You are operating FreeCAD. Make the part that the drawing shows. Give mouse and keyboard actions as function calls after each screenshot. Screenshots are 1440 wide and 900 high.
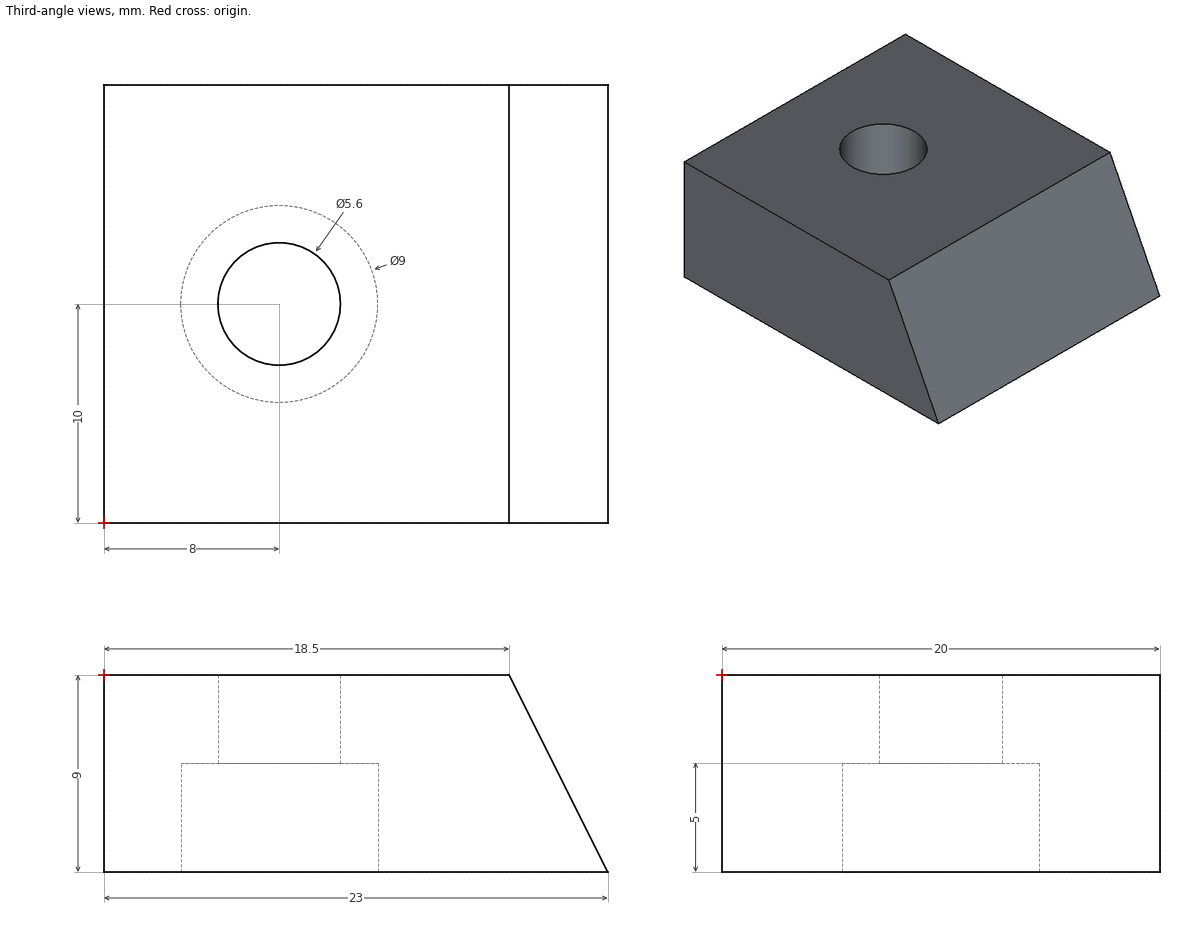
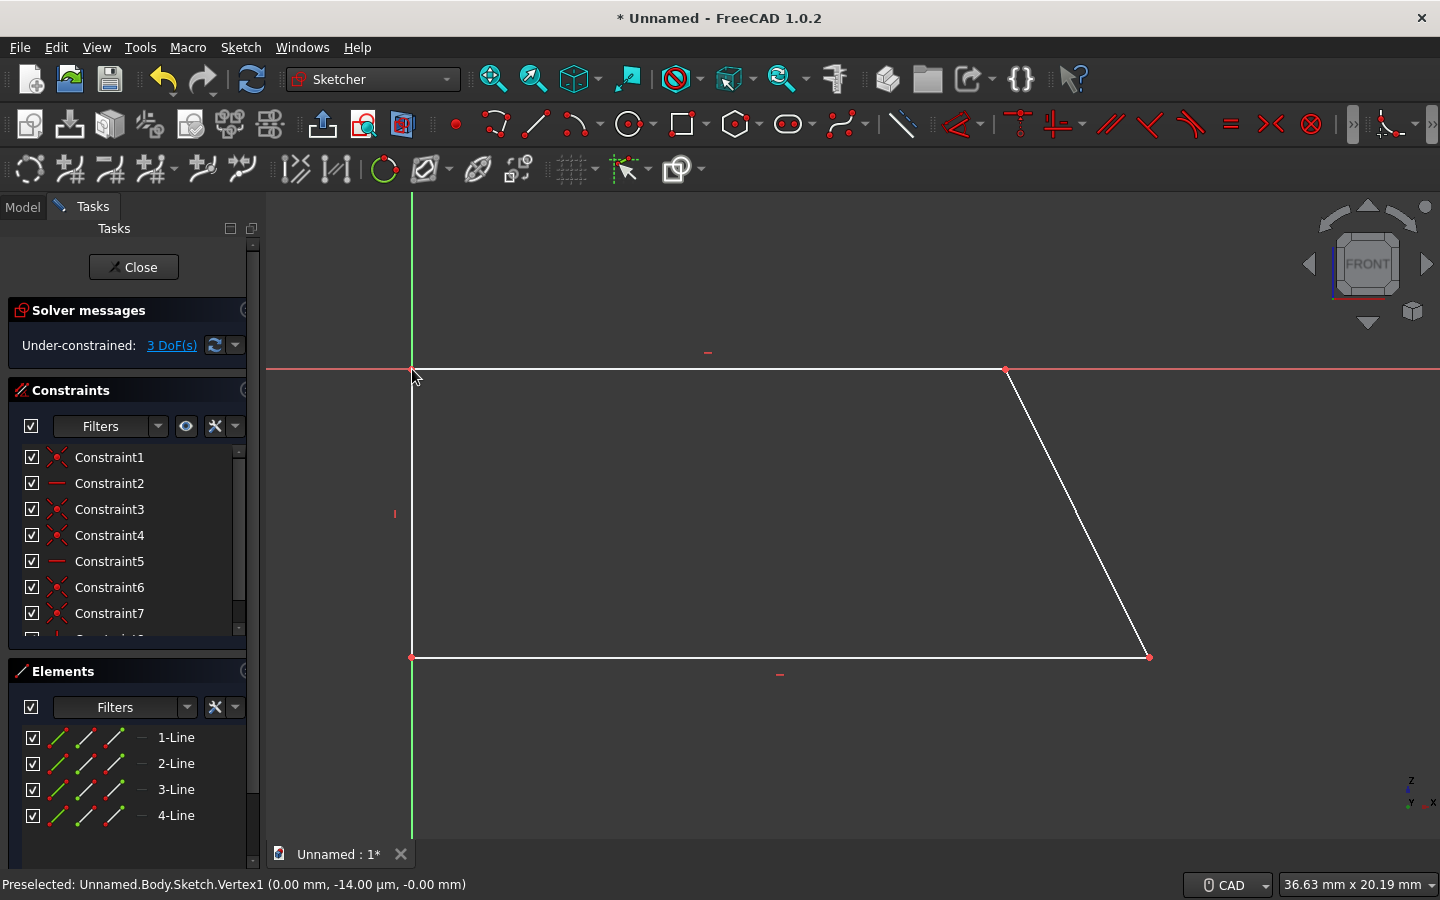
key(d)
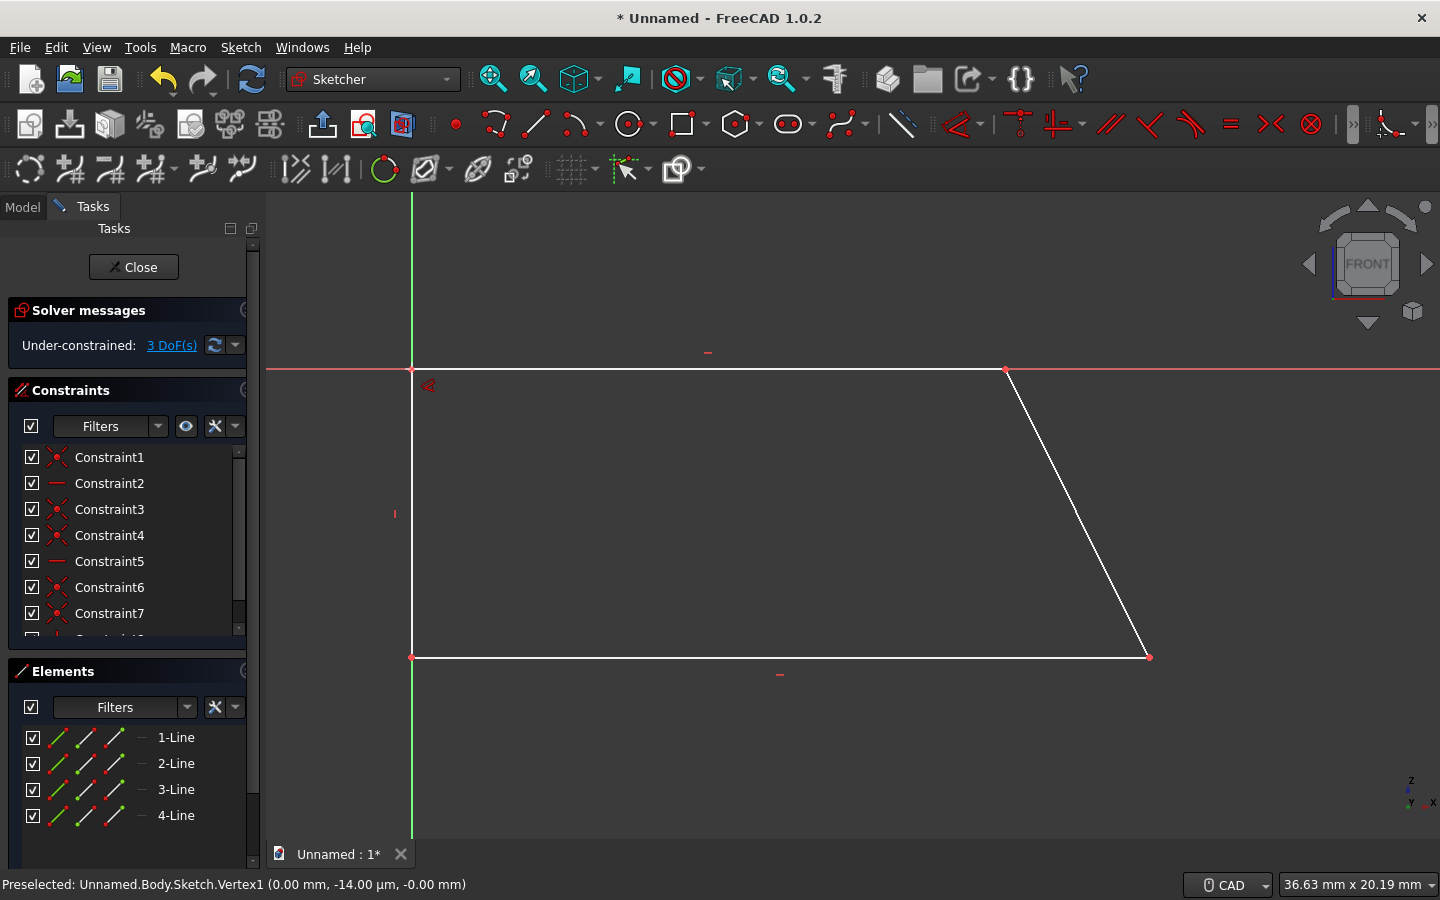
click(412, 571)
click(378, 514)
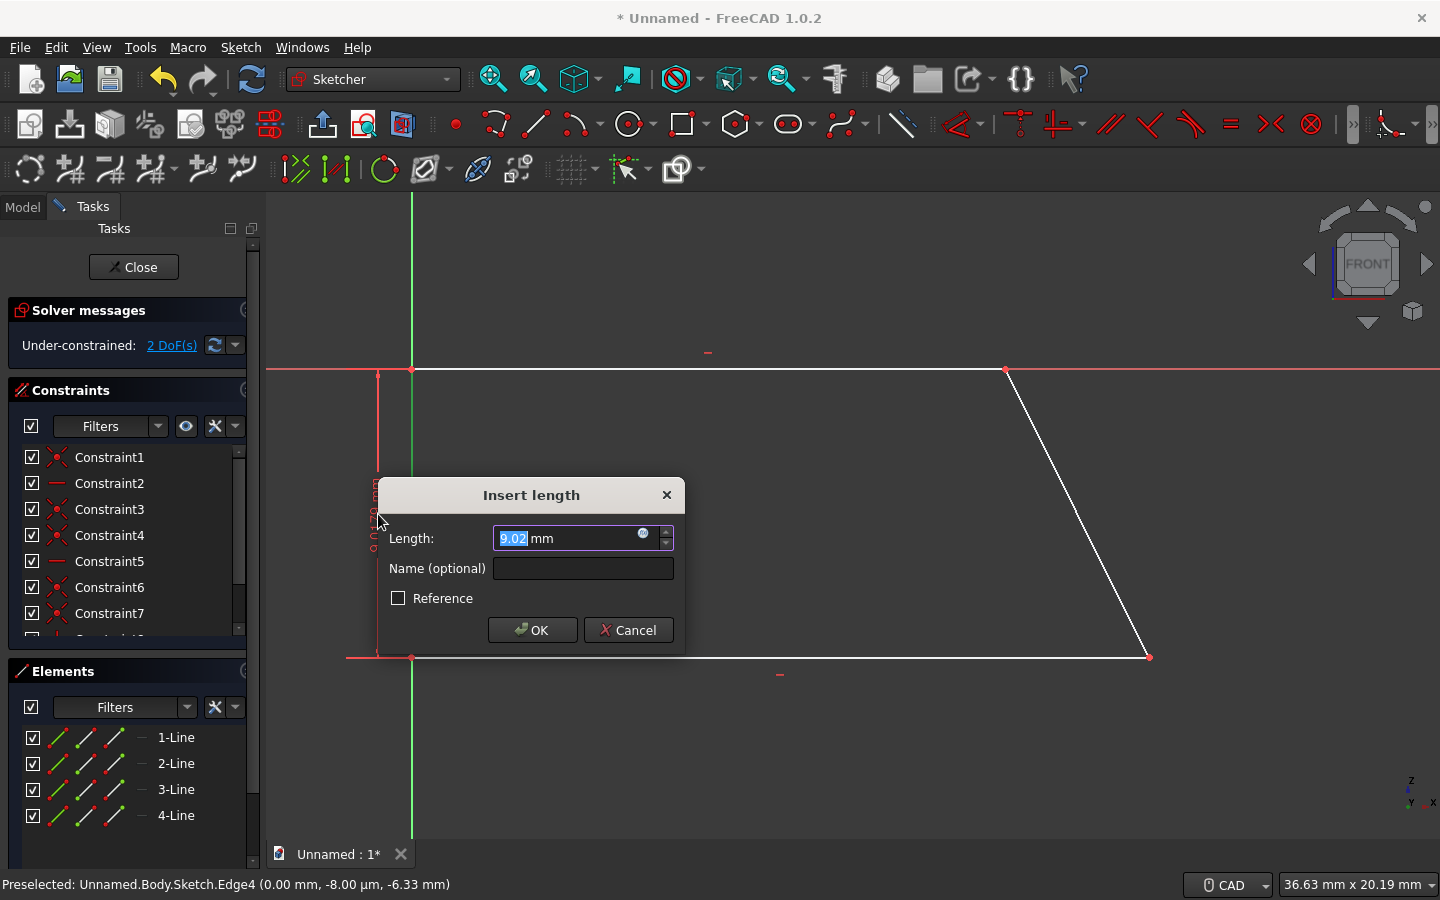
text(9)
key(Return)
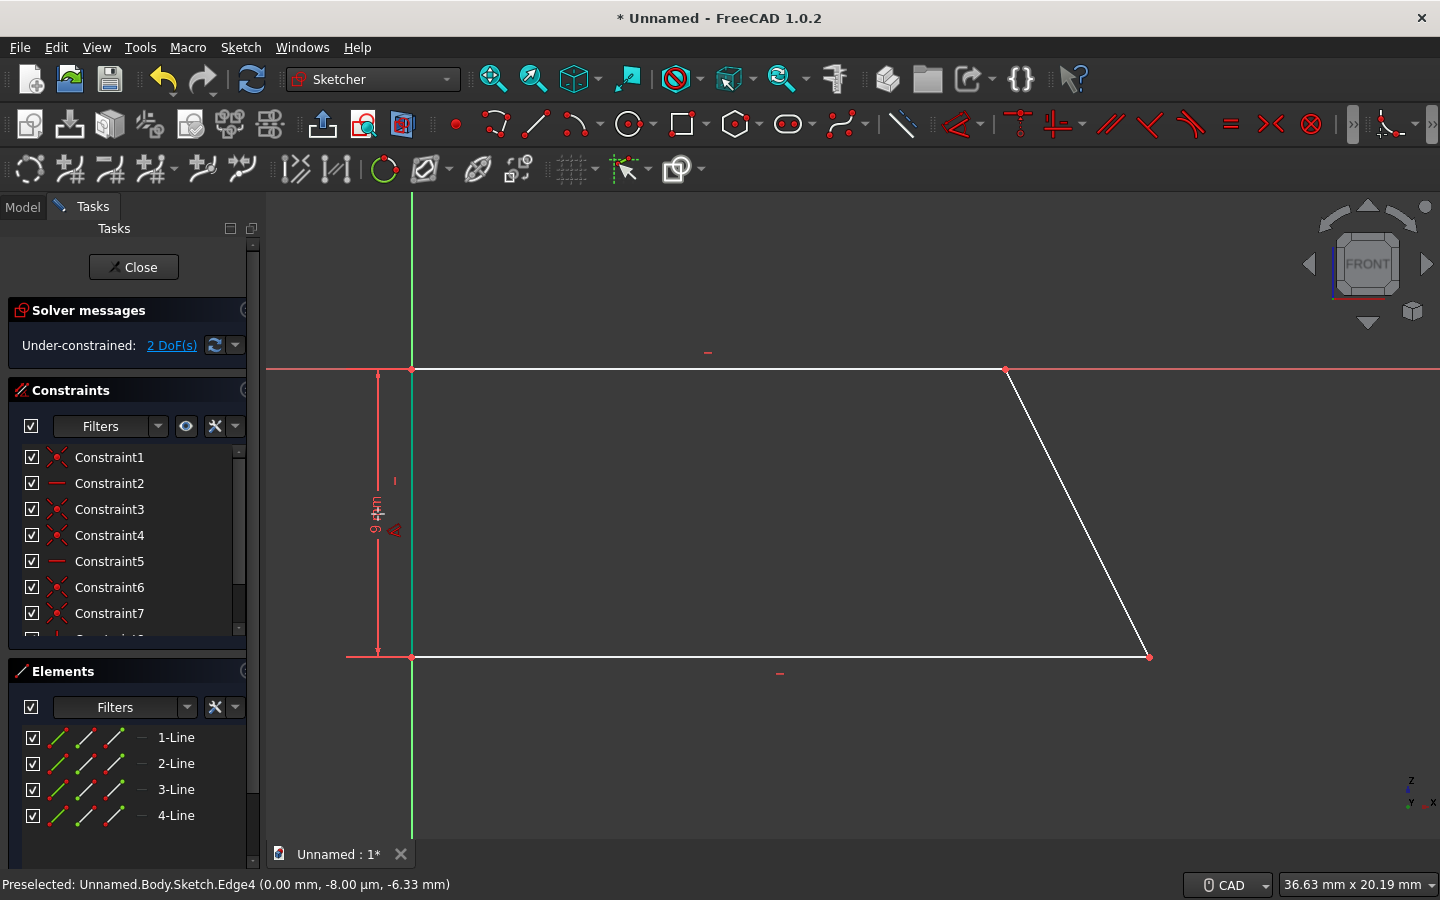
click(928, 657)
click(780, 691)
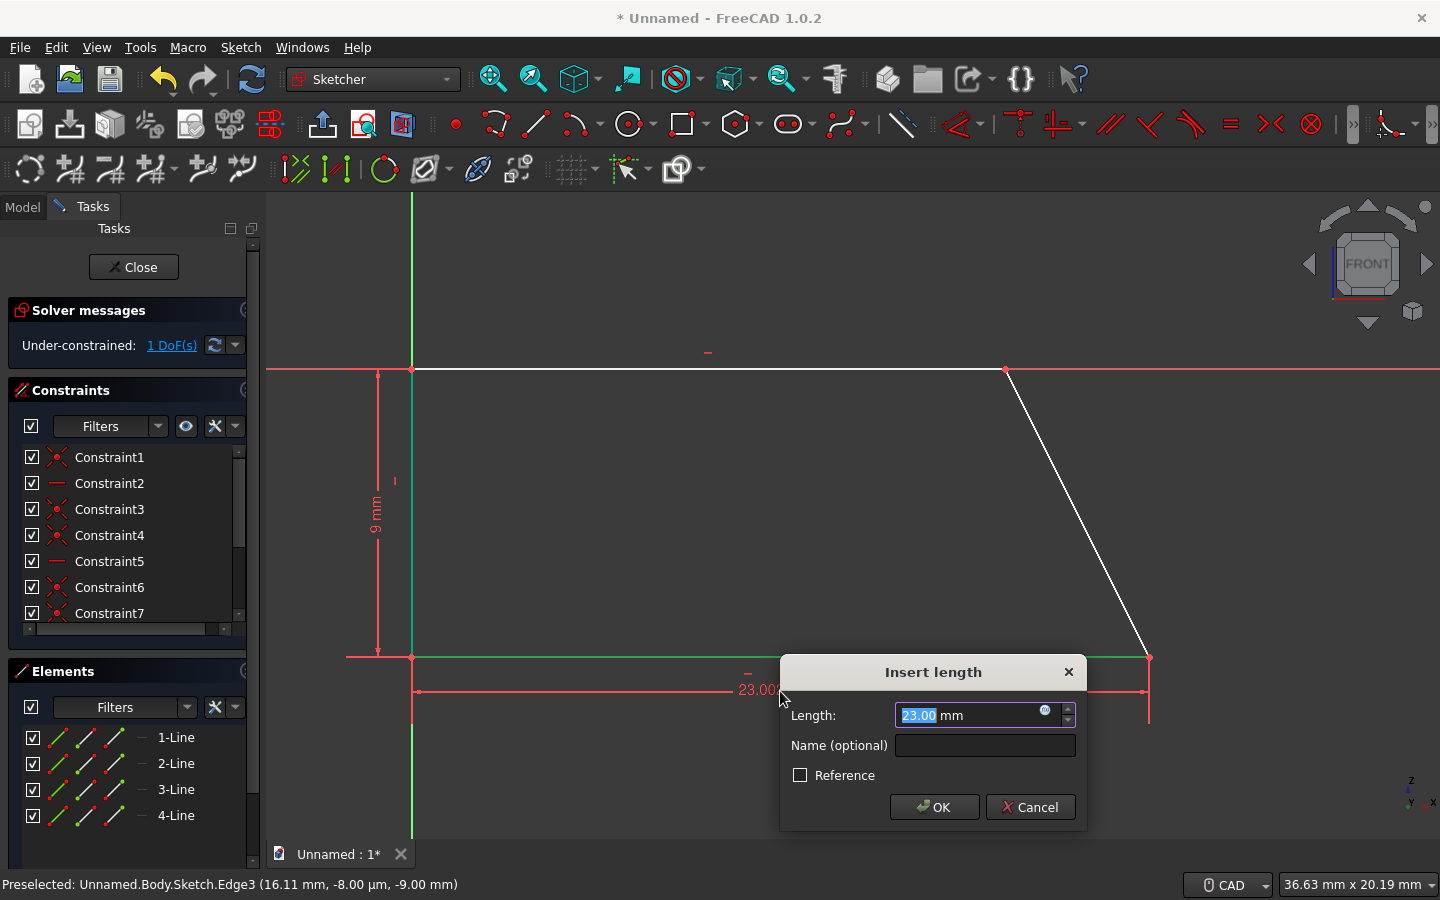
text(23)
key(Return)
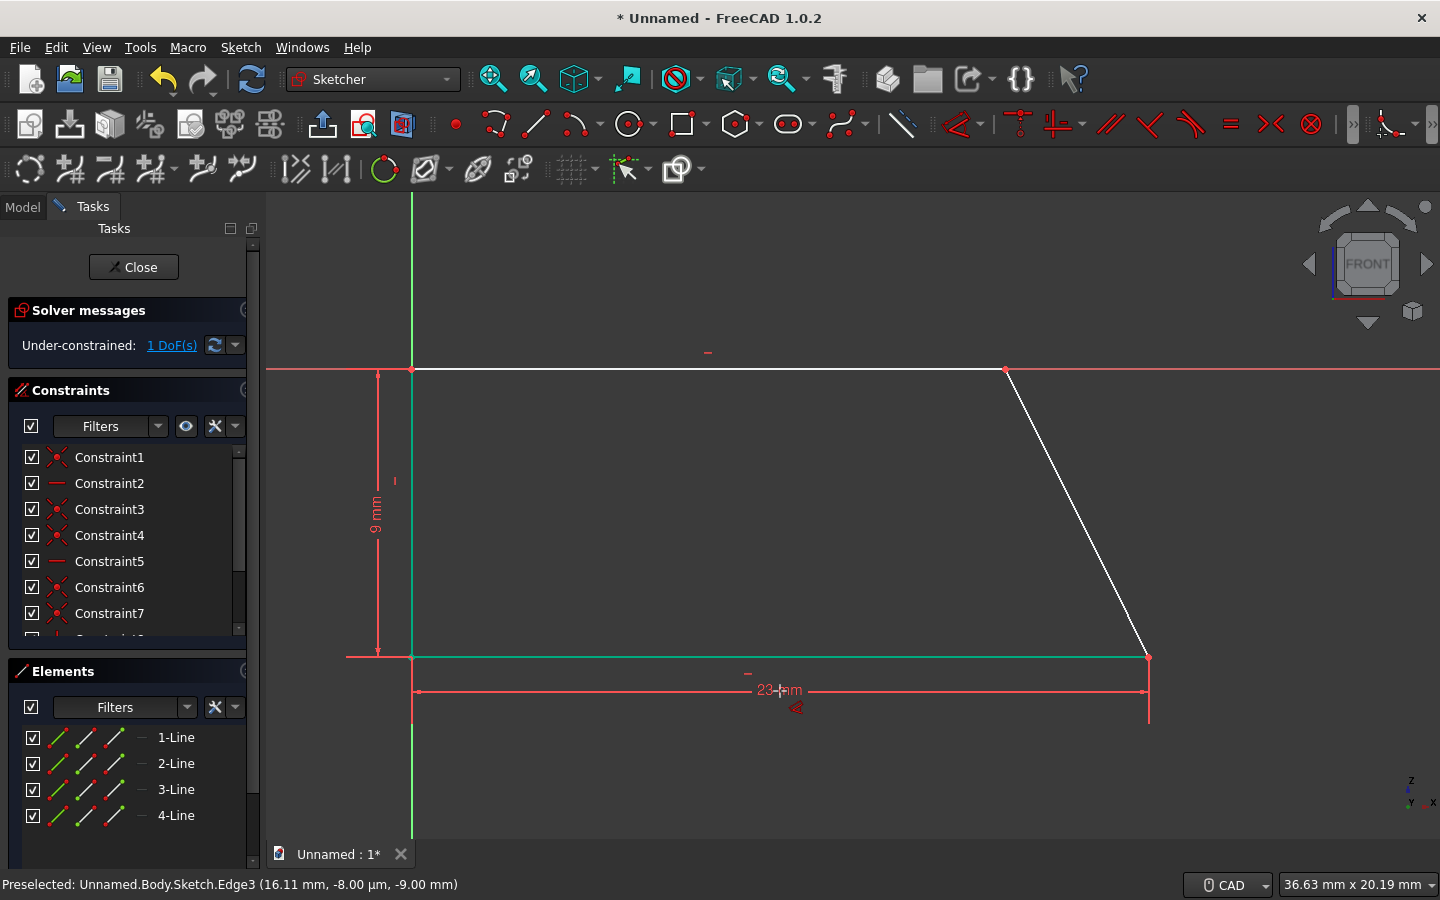
click(590, 369)
click(708, 335)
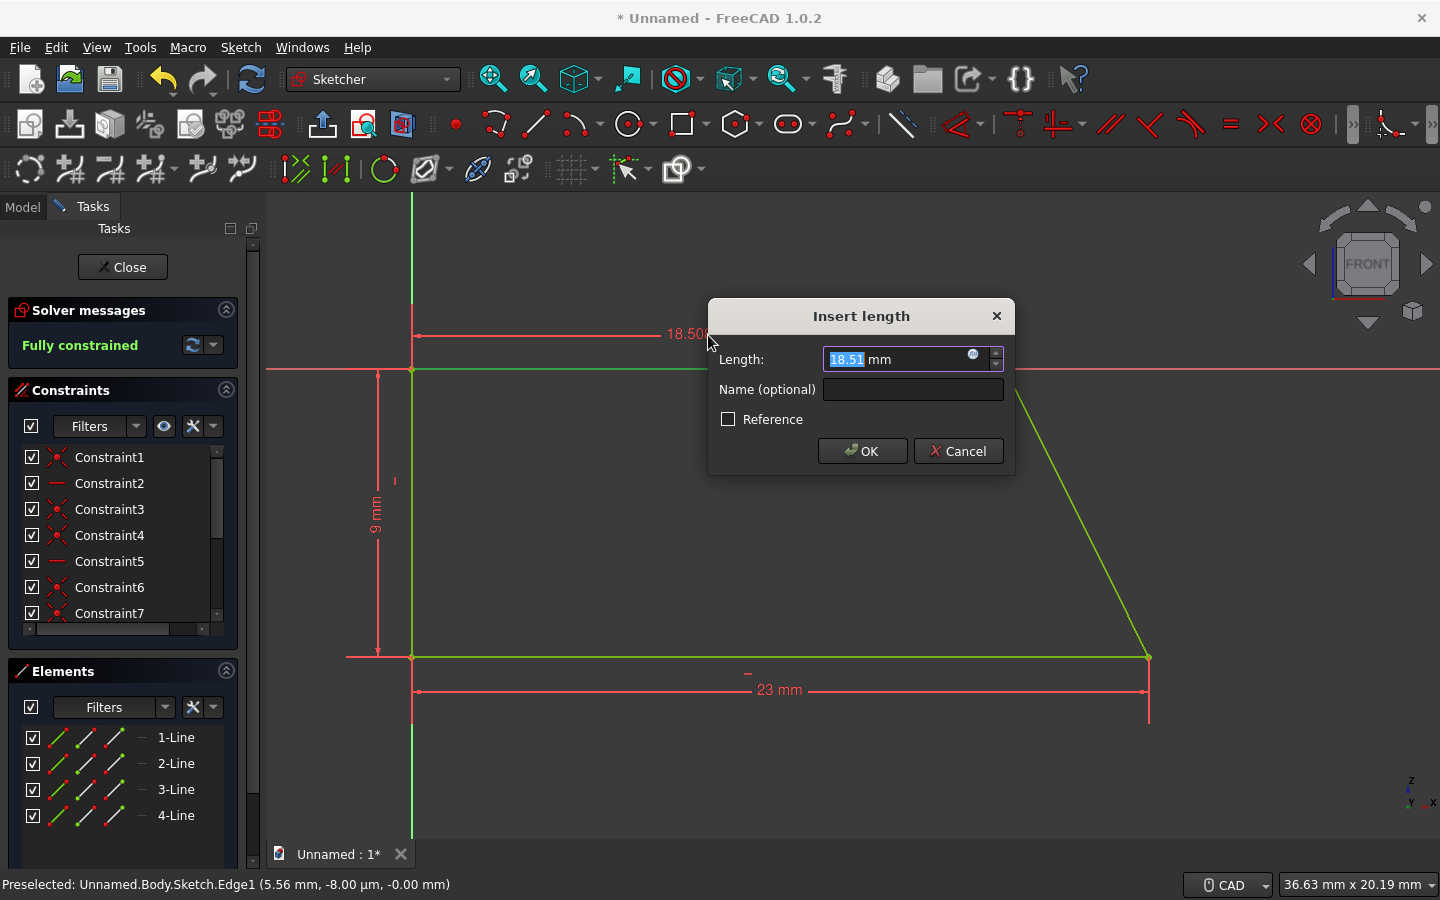
text(18.5)
key(Return)
key(Escape)